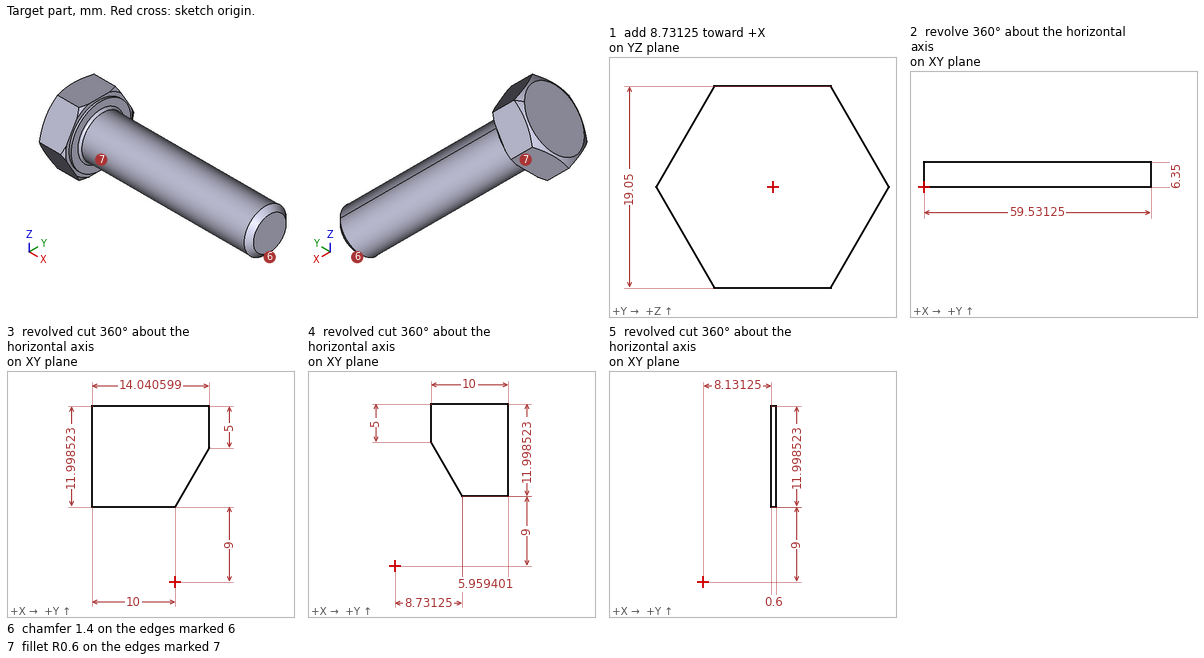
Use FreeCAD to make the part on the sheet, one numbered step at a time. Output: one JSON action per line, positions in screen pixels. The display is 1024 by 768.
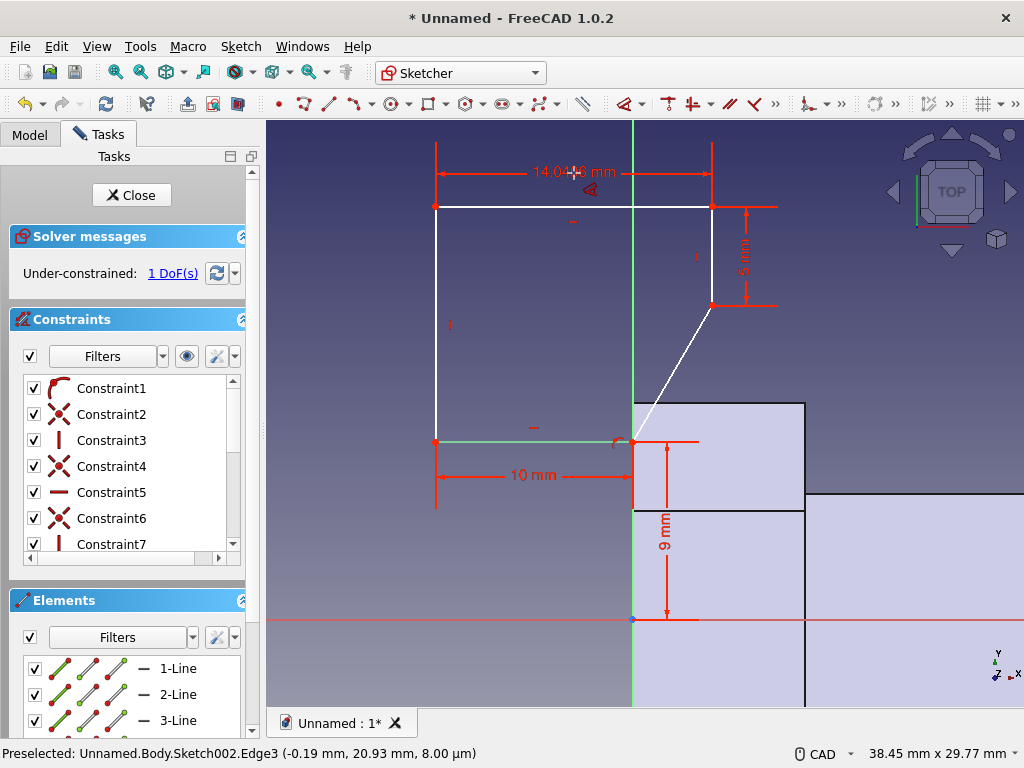
{"action": "left_click", "coordinate": [436, 278]}
{"action": "left_click", "coordinate": [402, 325]}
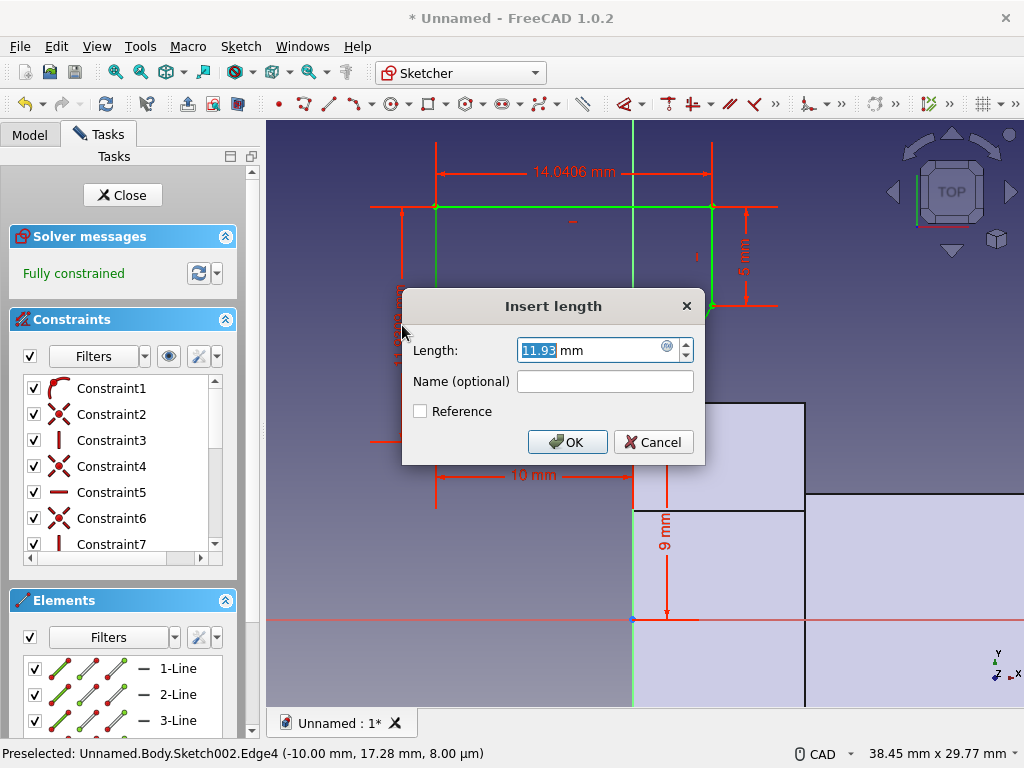
{"action": "type", "text": "11.998523"}
{"action": "key", "text": "Return"}
{"action": "key", "text": "Escape"}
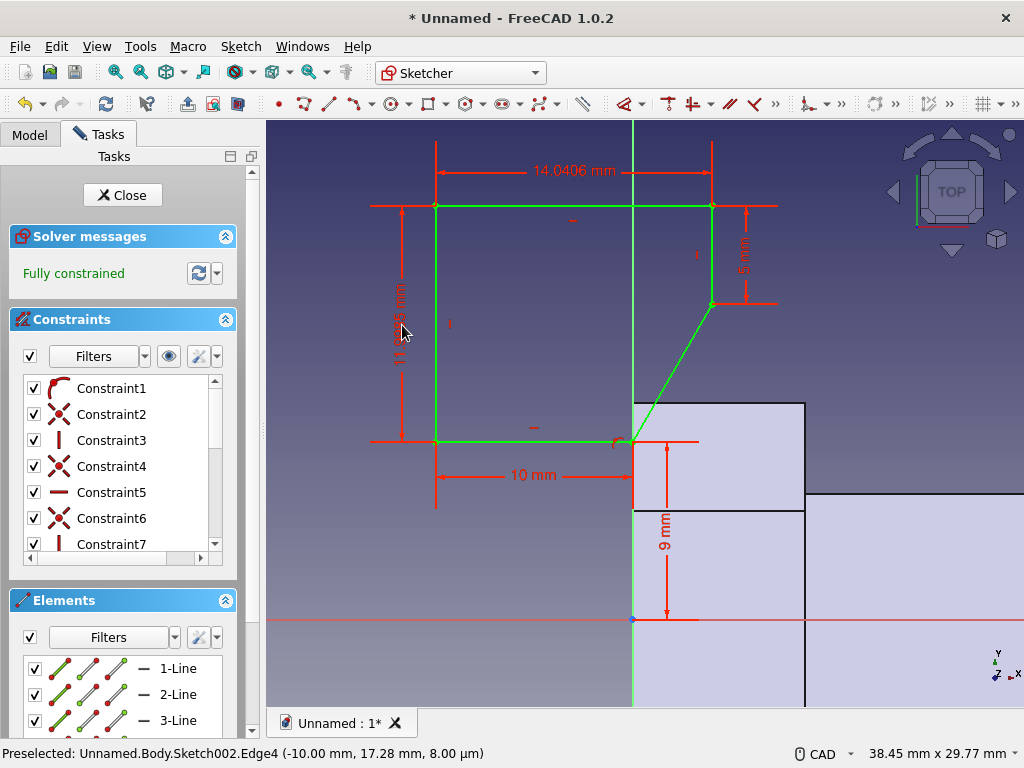
{"action": "left_click", "coordinate": [123, 195]}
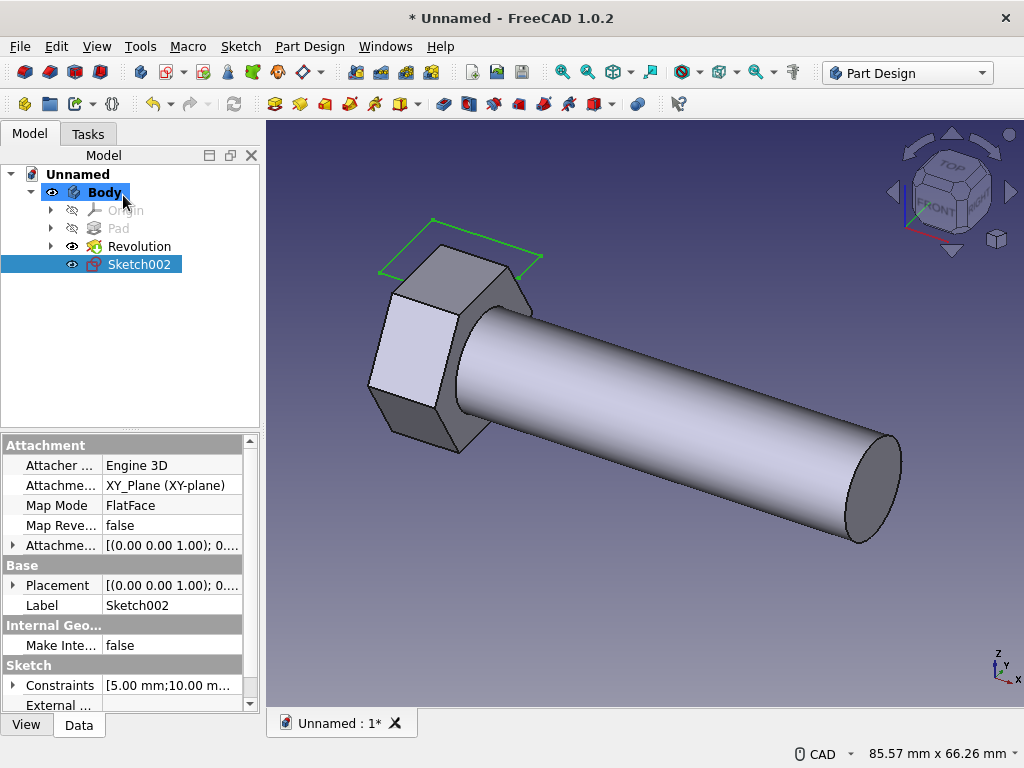
{"action": "left_click", "coordinate": [494, 104]}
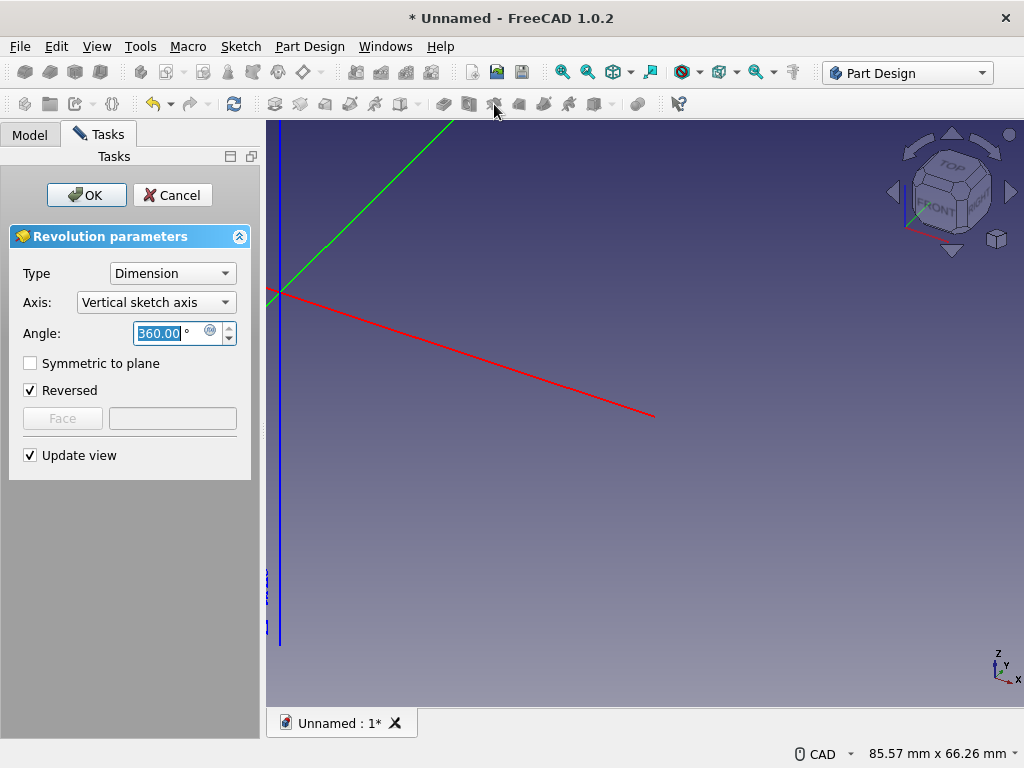
{"action": "left_click", "coordinate": [157, 302]}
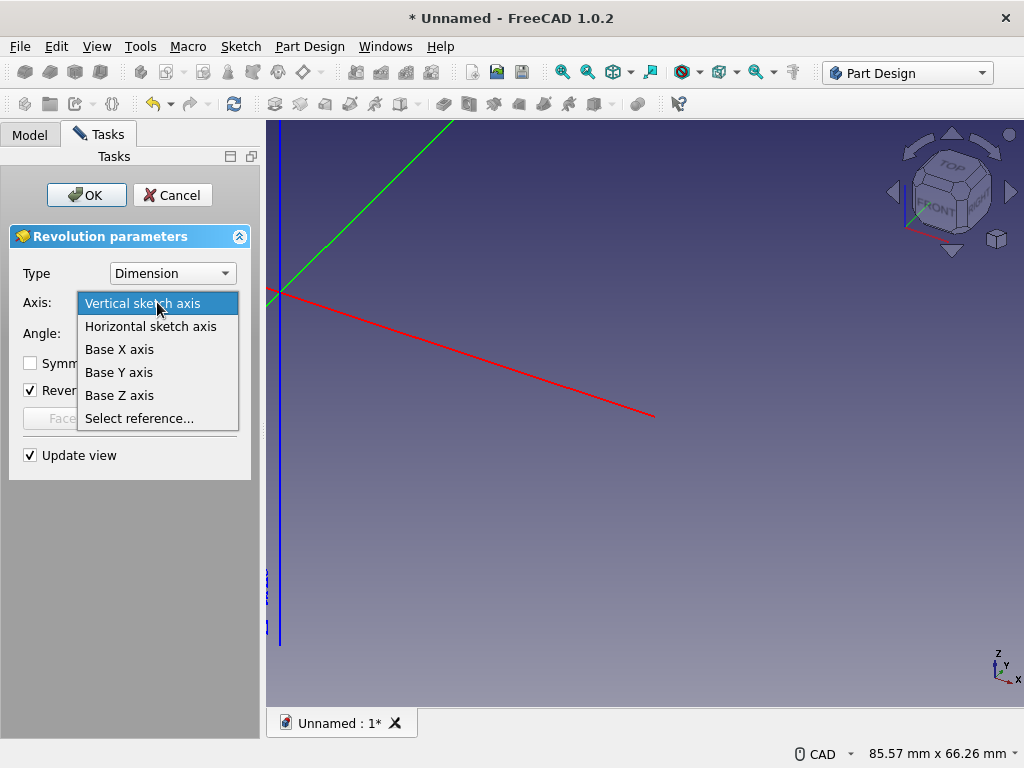
{"action": "left_click", "coordinate": [156, 326]}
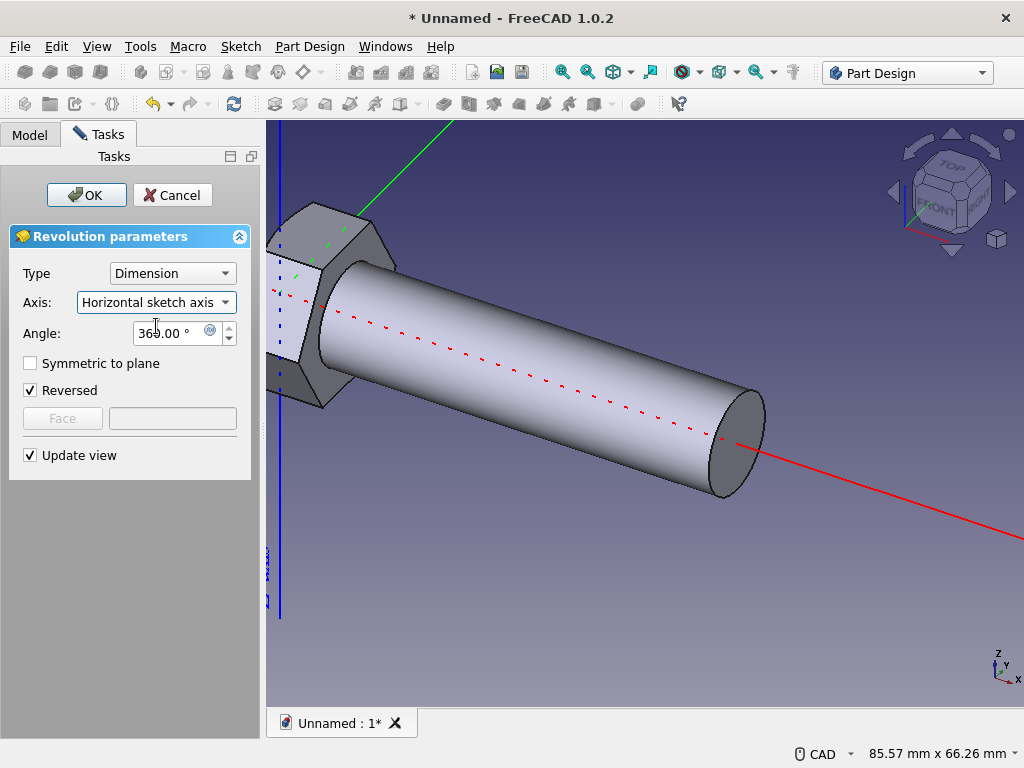
{"action": "left_click", "coordinate": [87, 195]}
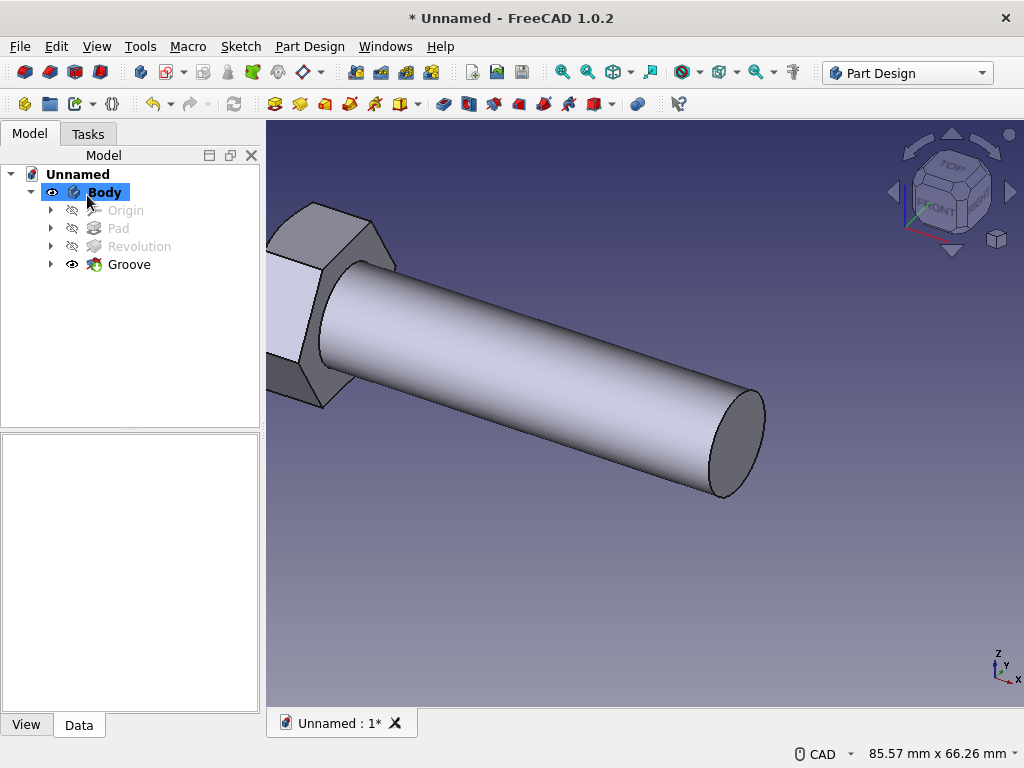
{"action": "left_click", "coordinate": [563, 72]}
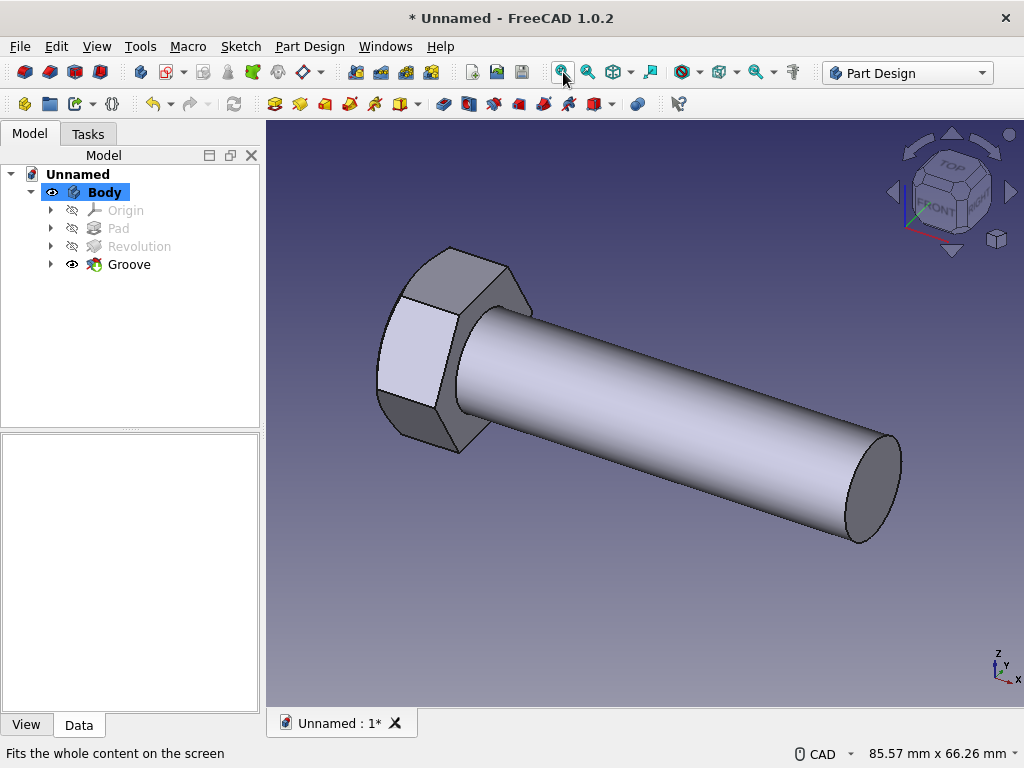
{"action": "left_click", "coordinate": [166, 72]}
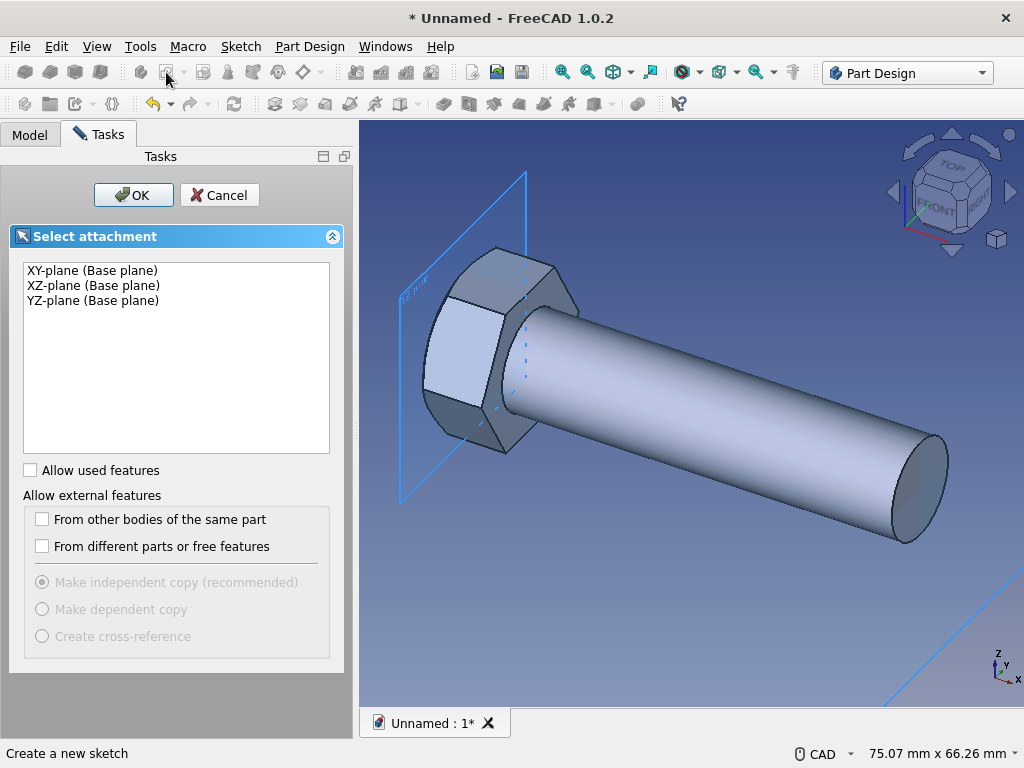
{"action": "left_click", "coordinate": [84, 270]}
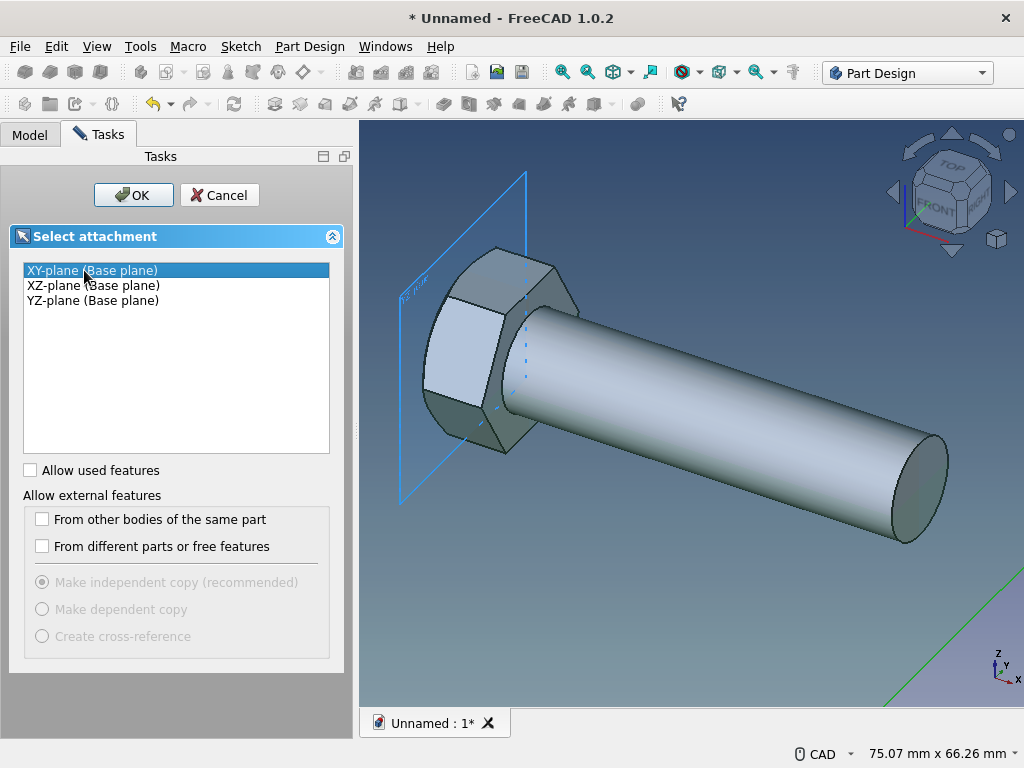
{"action": "left_click", "coordinate": [134, 195]}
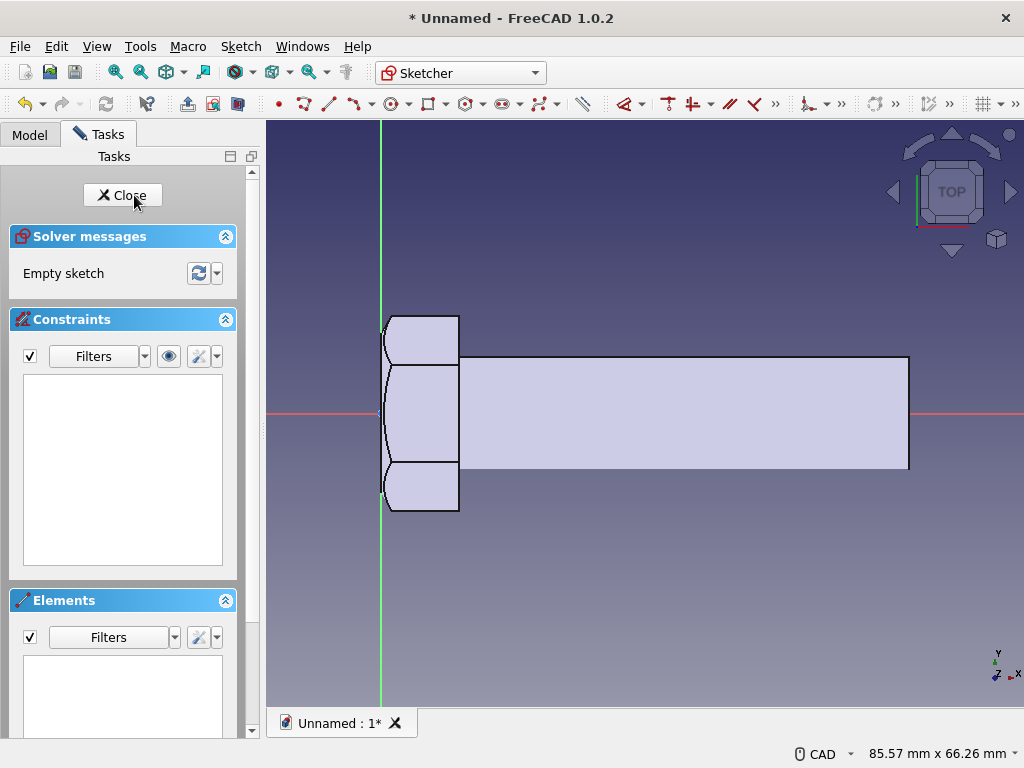
{"action": "left_click", "coordinate": [238, 104]}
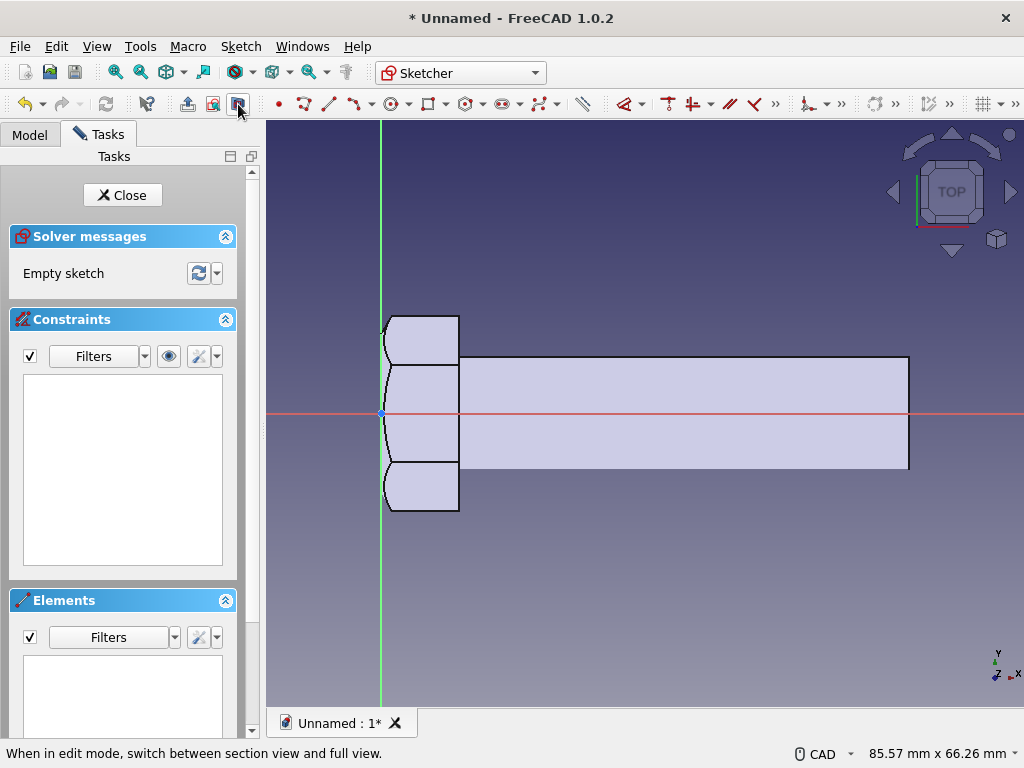
{"action": "scroll", "coordinate": [340, 245], "scroll_direction": "up", "scroll_amount": 4}